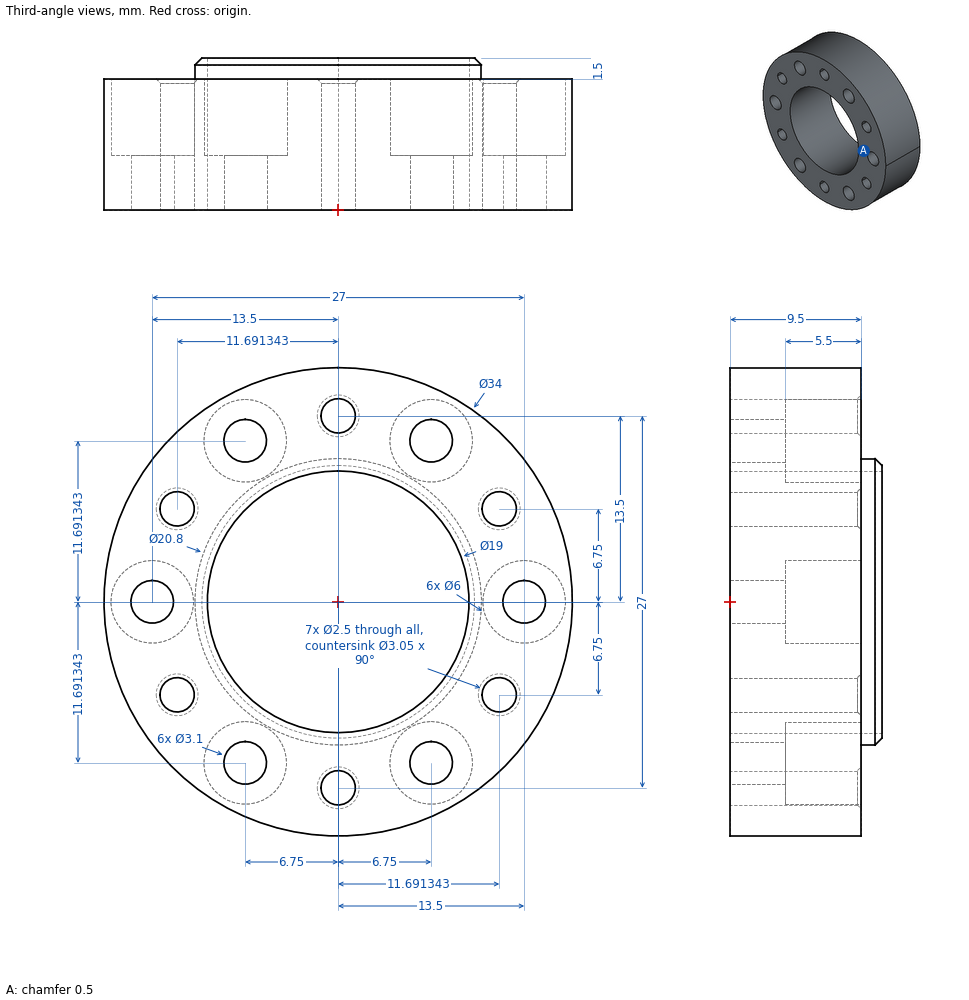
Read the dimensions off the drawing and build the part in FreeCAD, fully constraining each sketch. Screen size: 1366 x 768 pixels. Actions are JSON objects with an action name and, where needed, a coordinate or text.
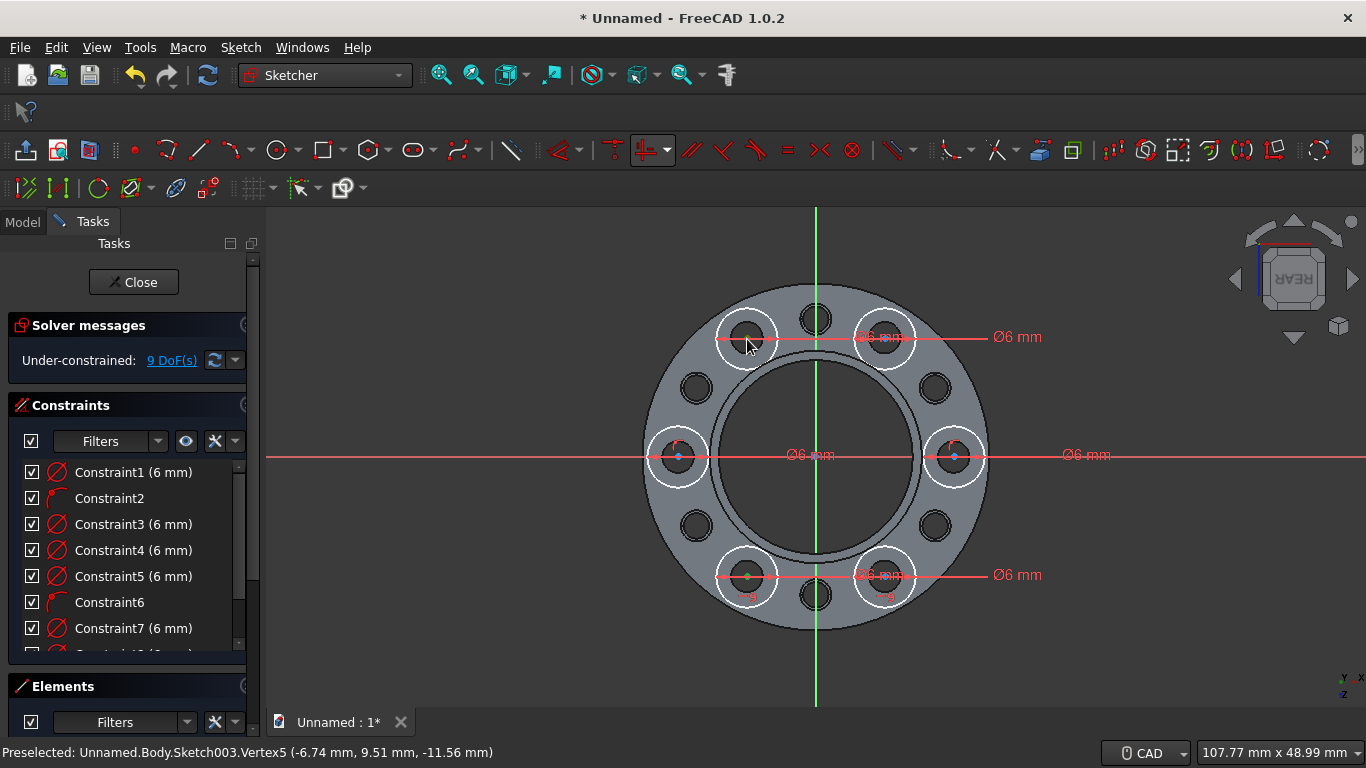
{"action": "left_click", "coordinate": [670, 150]}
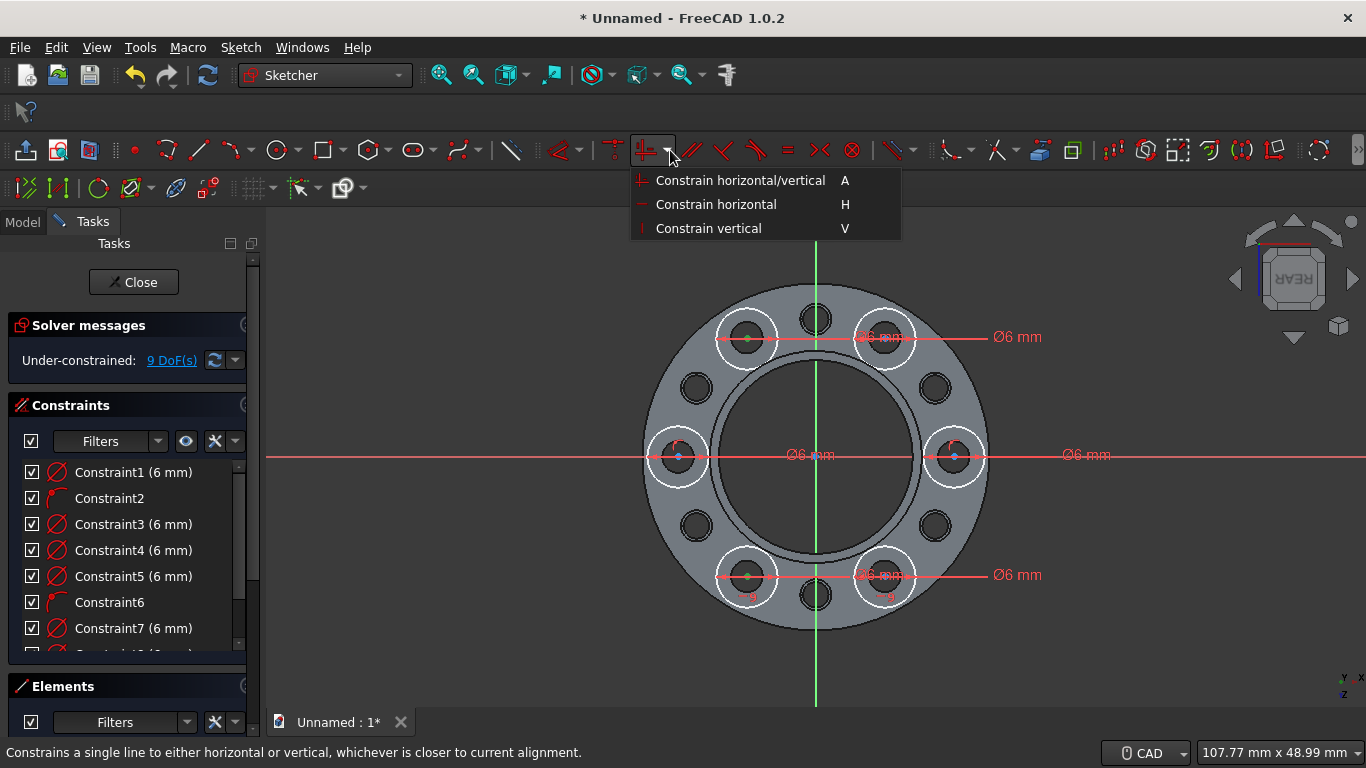
{"action": "left_click", "coordinate": [766, 228]}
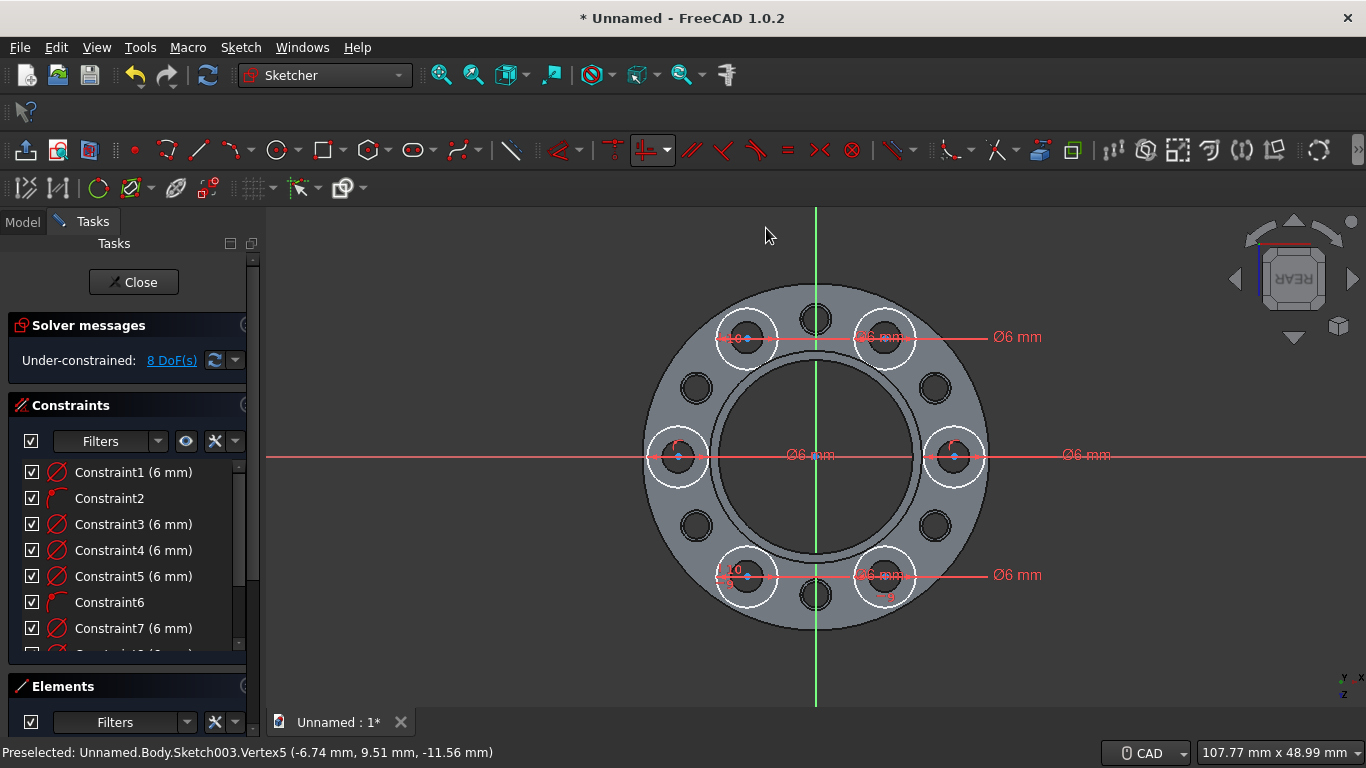
{"action": "left_click", "coordinate": [885, 577]}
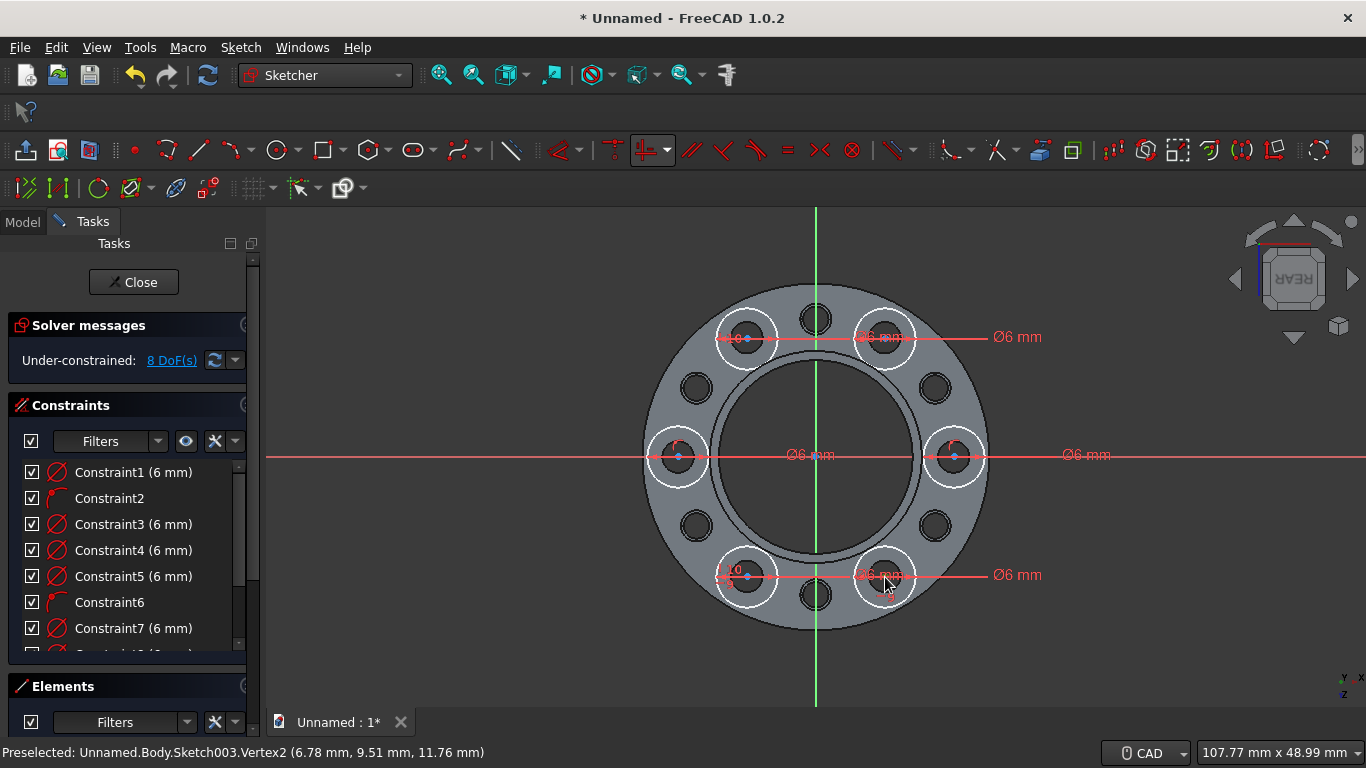
{"action": "left_click", "coordinate": [885, 339]}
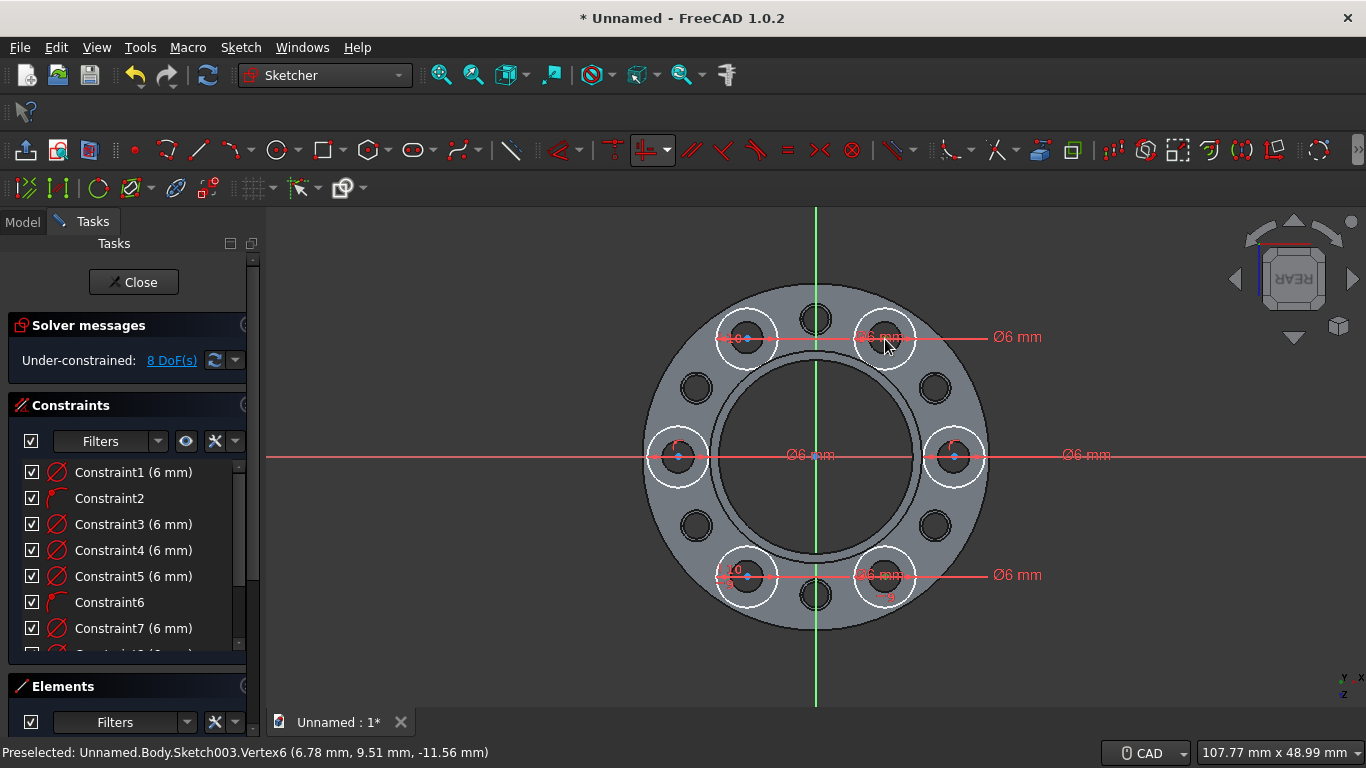
{"action": "left_click", "coordinate": [670, 150]}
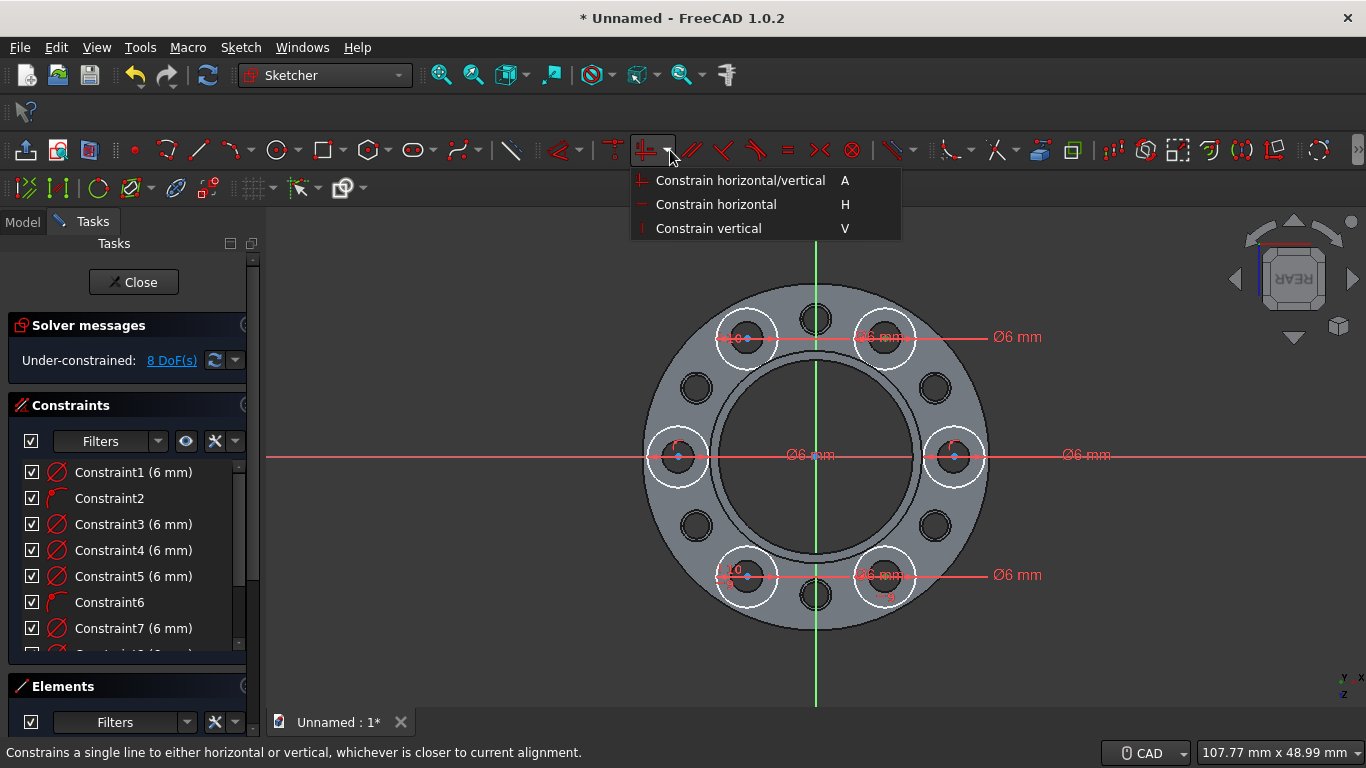
{"action": "left_click", "coordinate": [766, 228]}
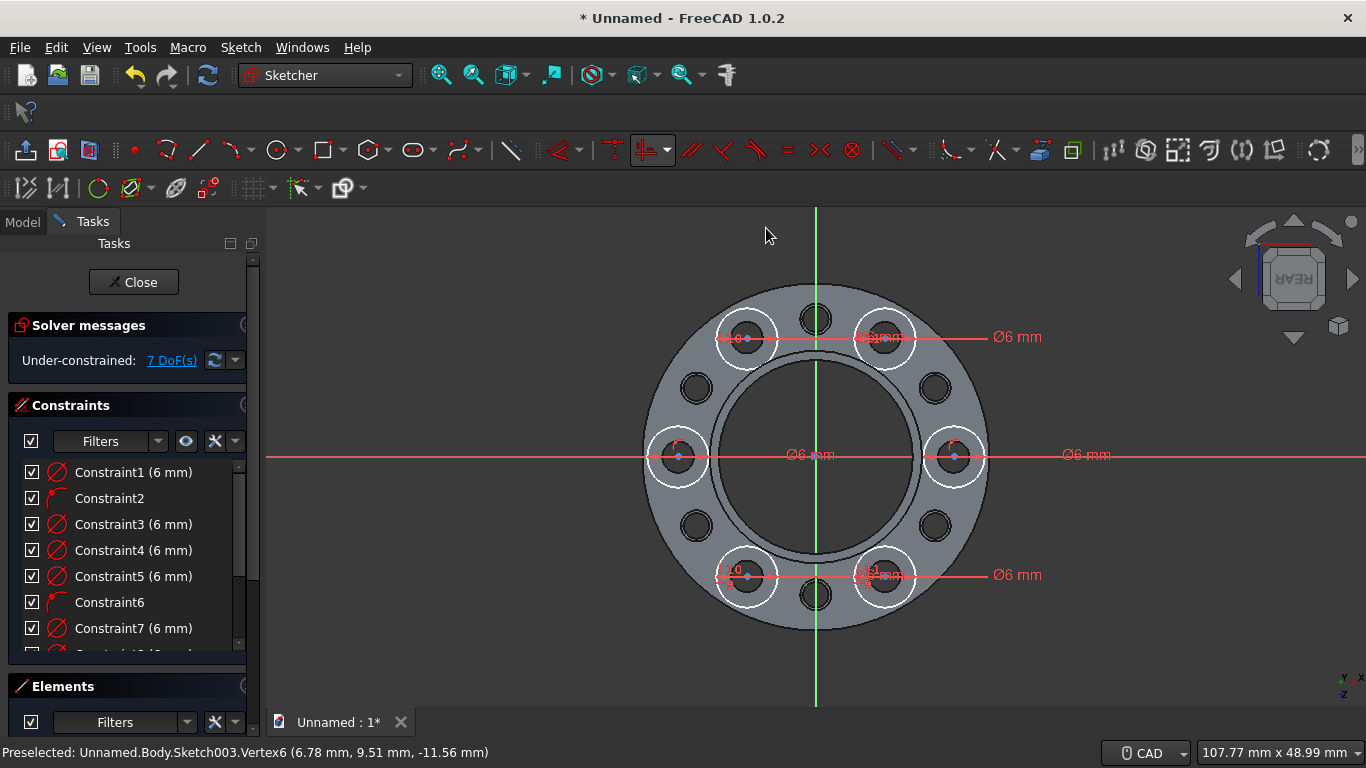
{"action": "left_click", "coordinate": [747, 339]}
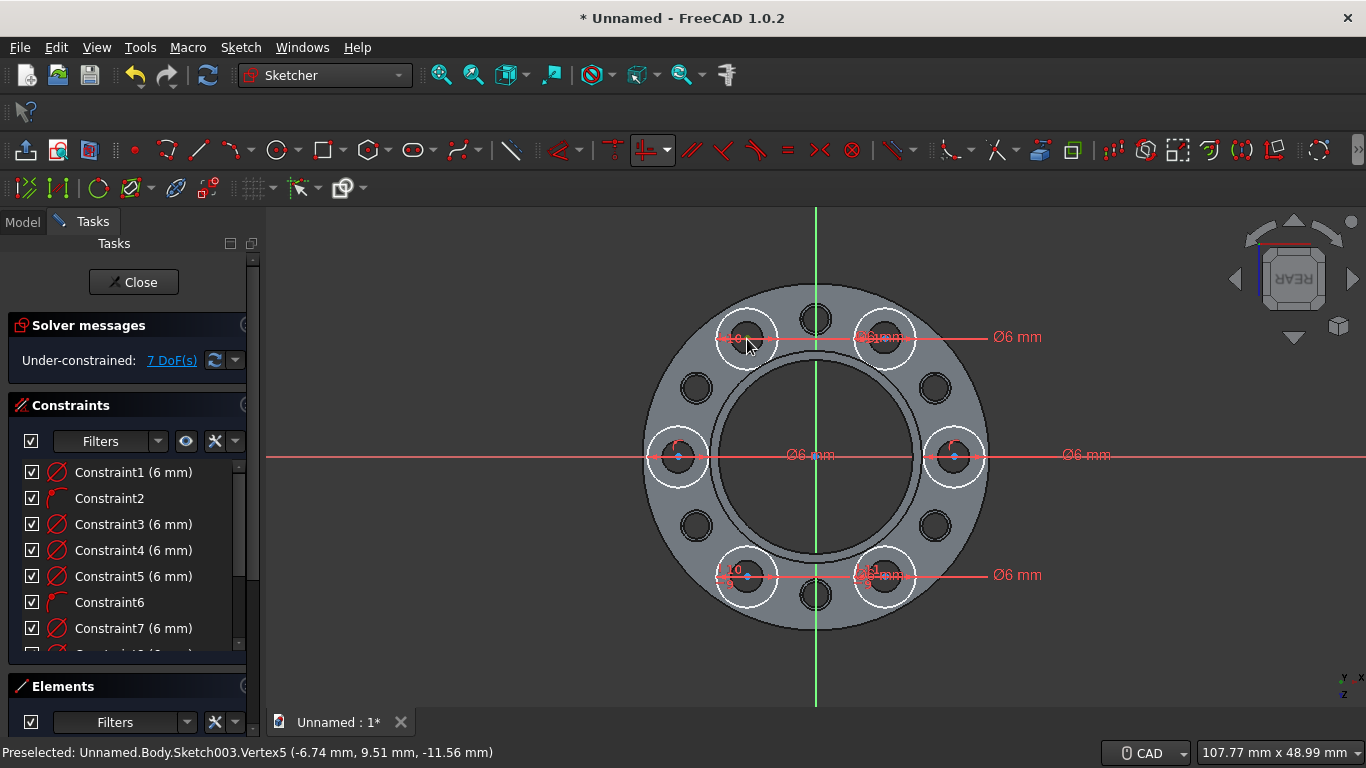
{"action": "left_click", "coordinate": [885, 339]}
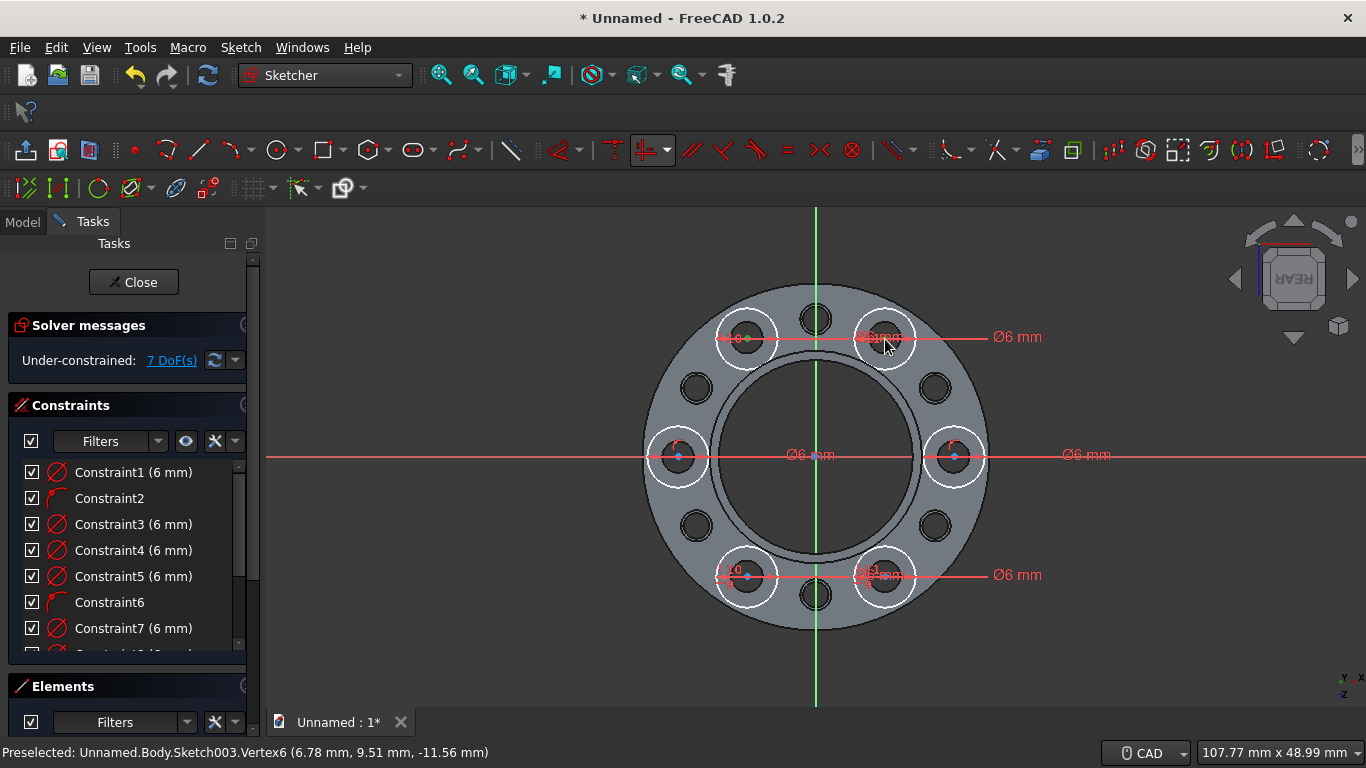
{"action": "left_click", "coordinate": [670, 150]}